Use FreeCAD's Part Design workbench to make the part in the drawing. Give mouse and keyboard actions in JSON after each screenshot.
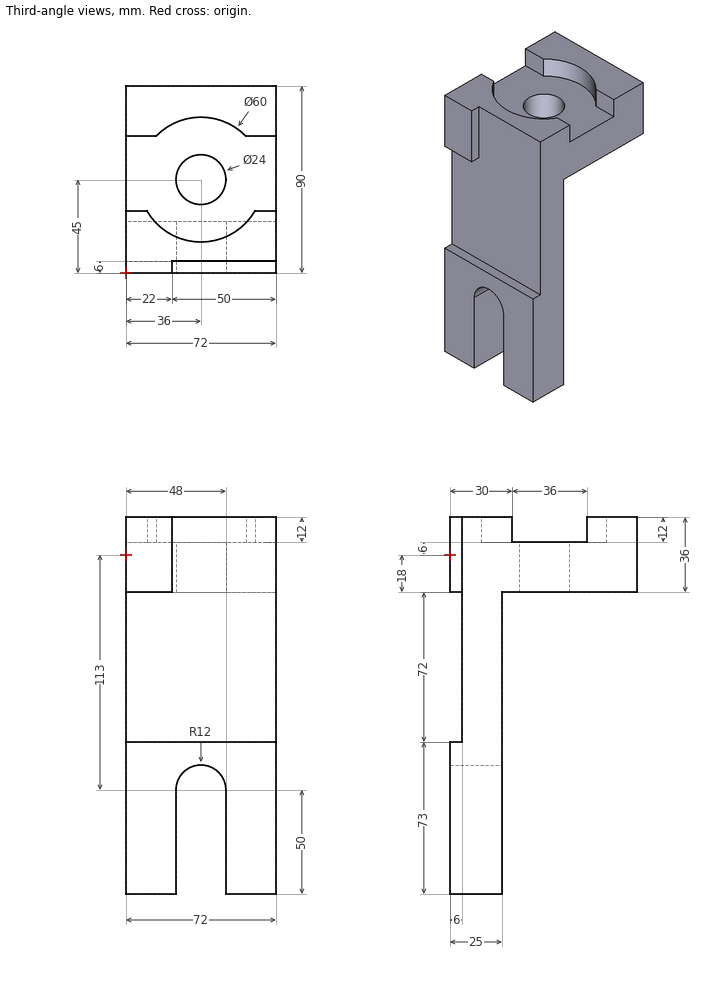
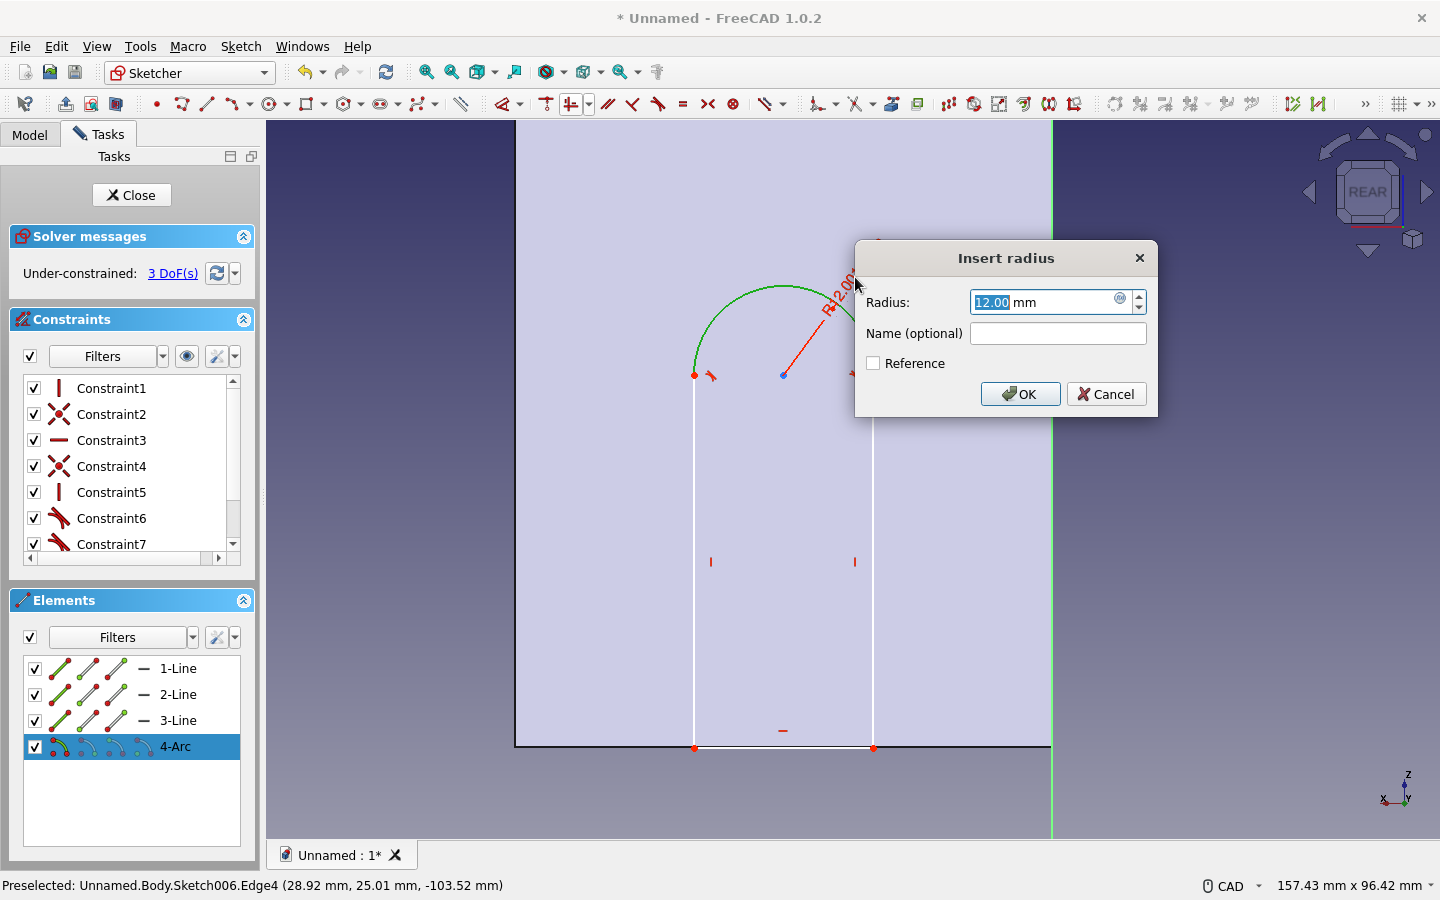
{"action": "type", "text": "12"}
{"action": "key", "text": "Return"}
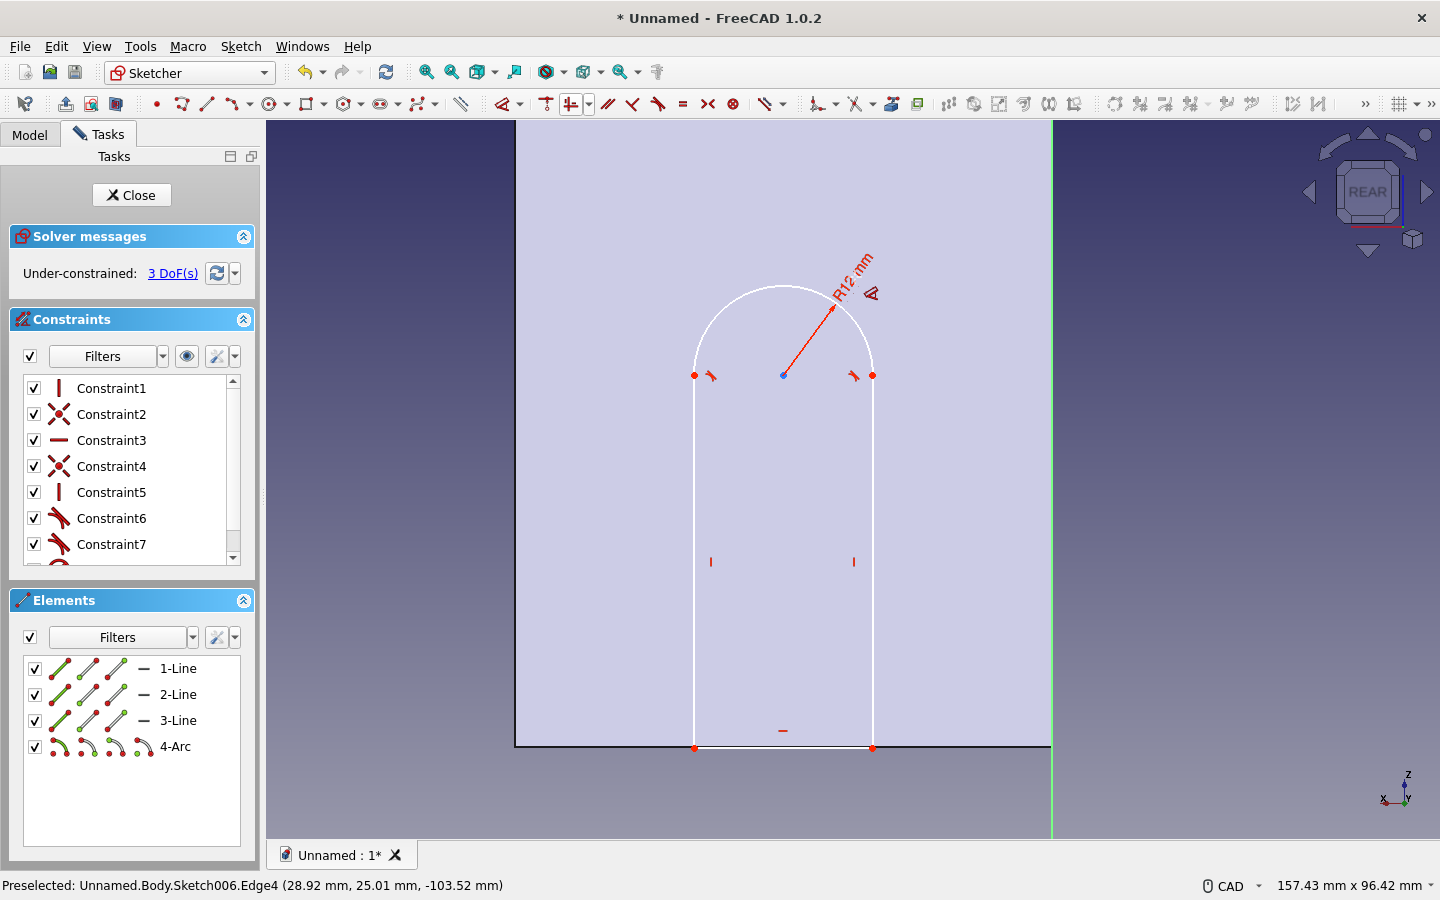
{"action": "left_click", "coordinate": [694, 487]}
{"action": "left_click", "coordinate": [660, 562]}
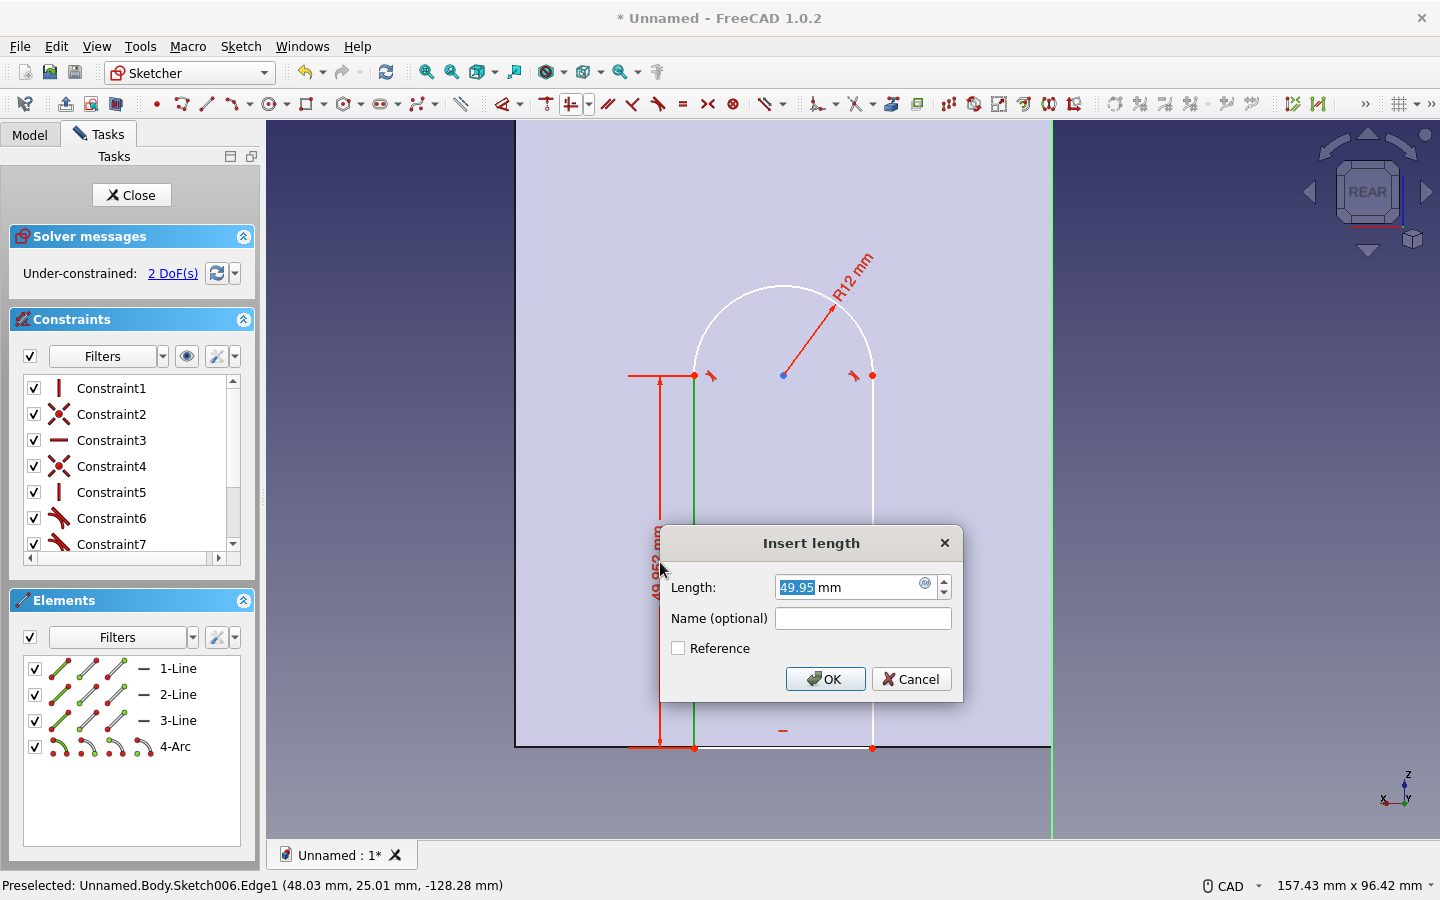
{"action": "type", "text": "50"}
{"action": "key", "text": "Return"}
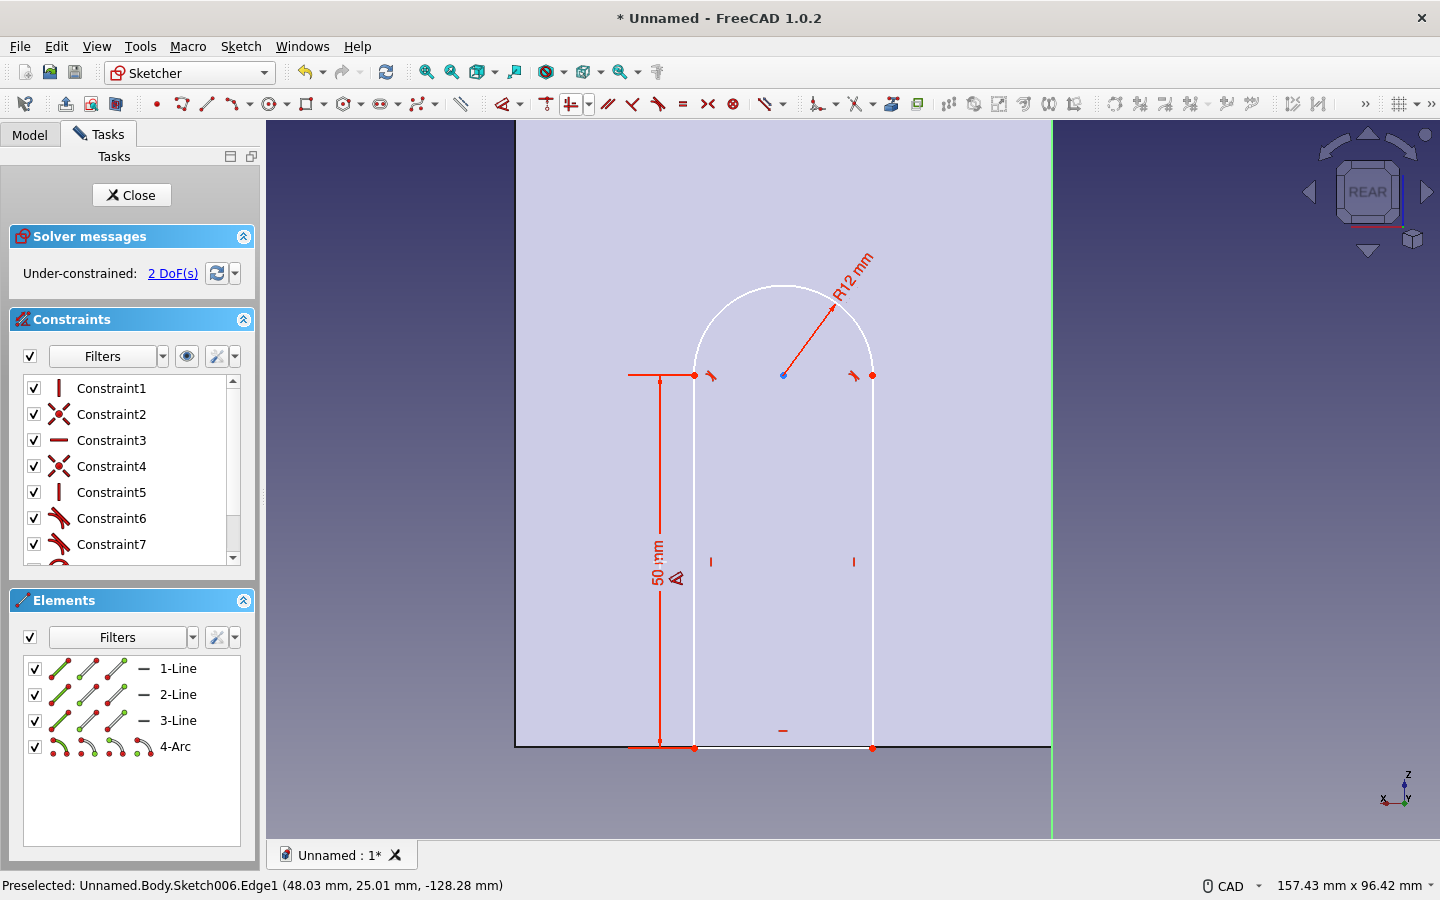
{"action": "left_click", "coordinate": [694, 375]}
{"action": "left_click", "coordinate": [791, 409]}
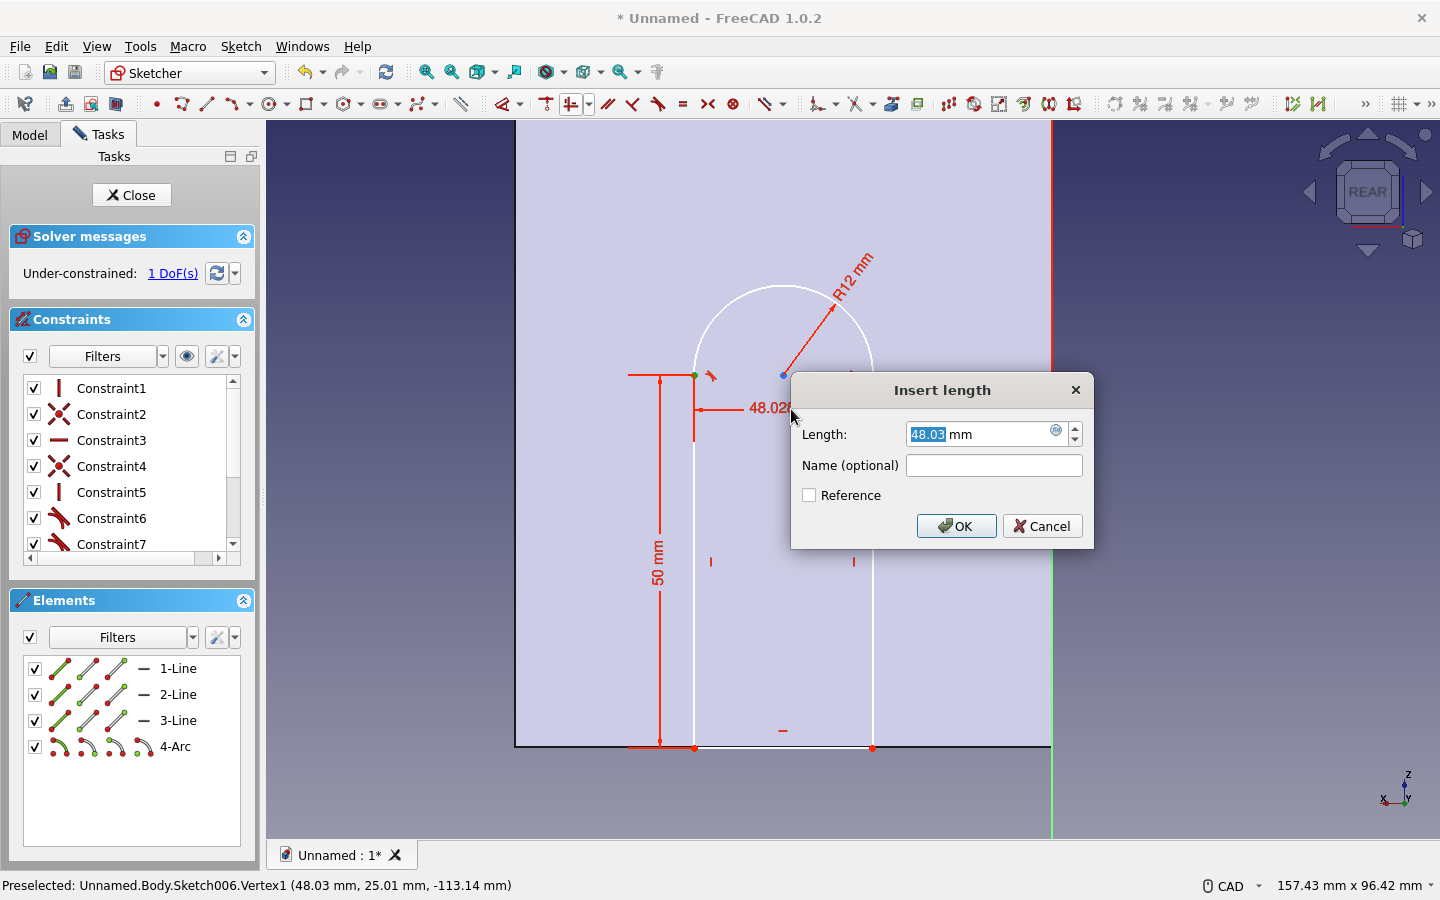
{"action": "type", "text": "48"}
{"action": "key", "text": "Return"}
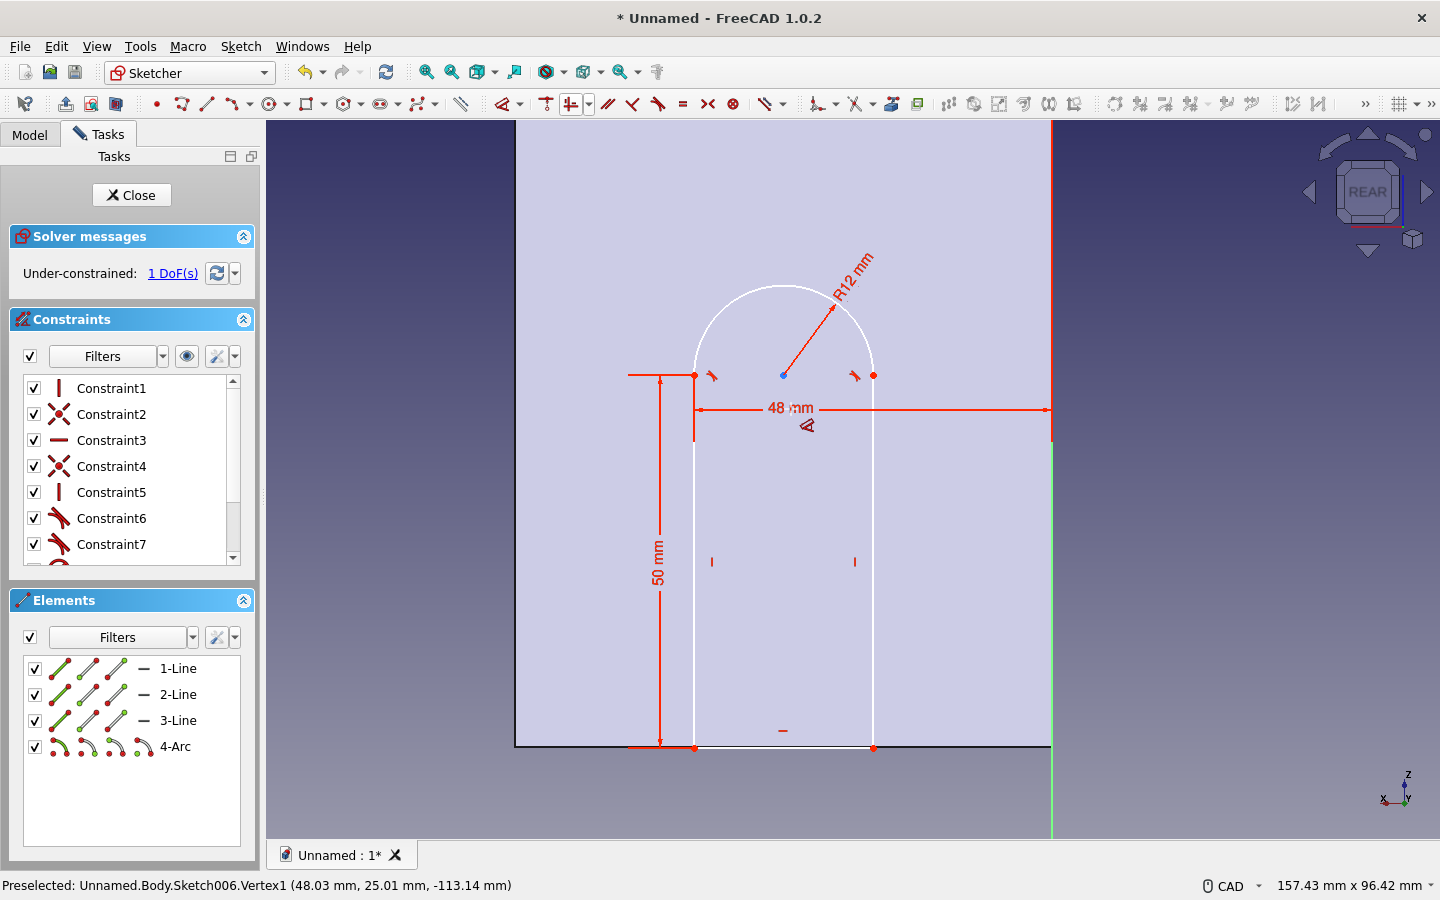
{"action": "left_click", "coordinate": [694, 375]}
{"action": "left_click", "coordinate": [1086, 262]}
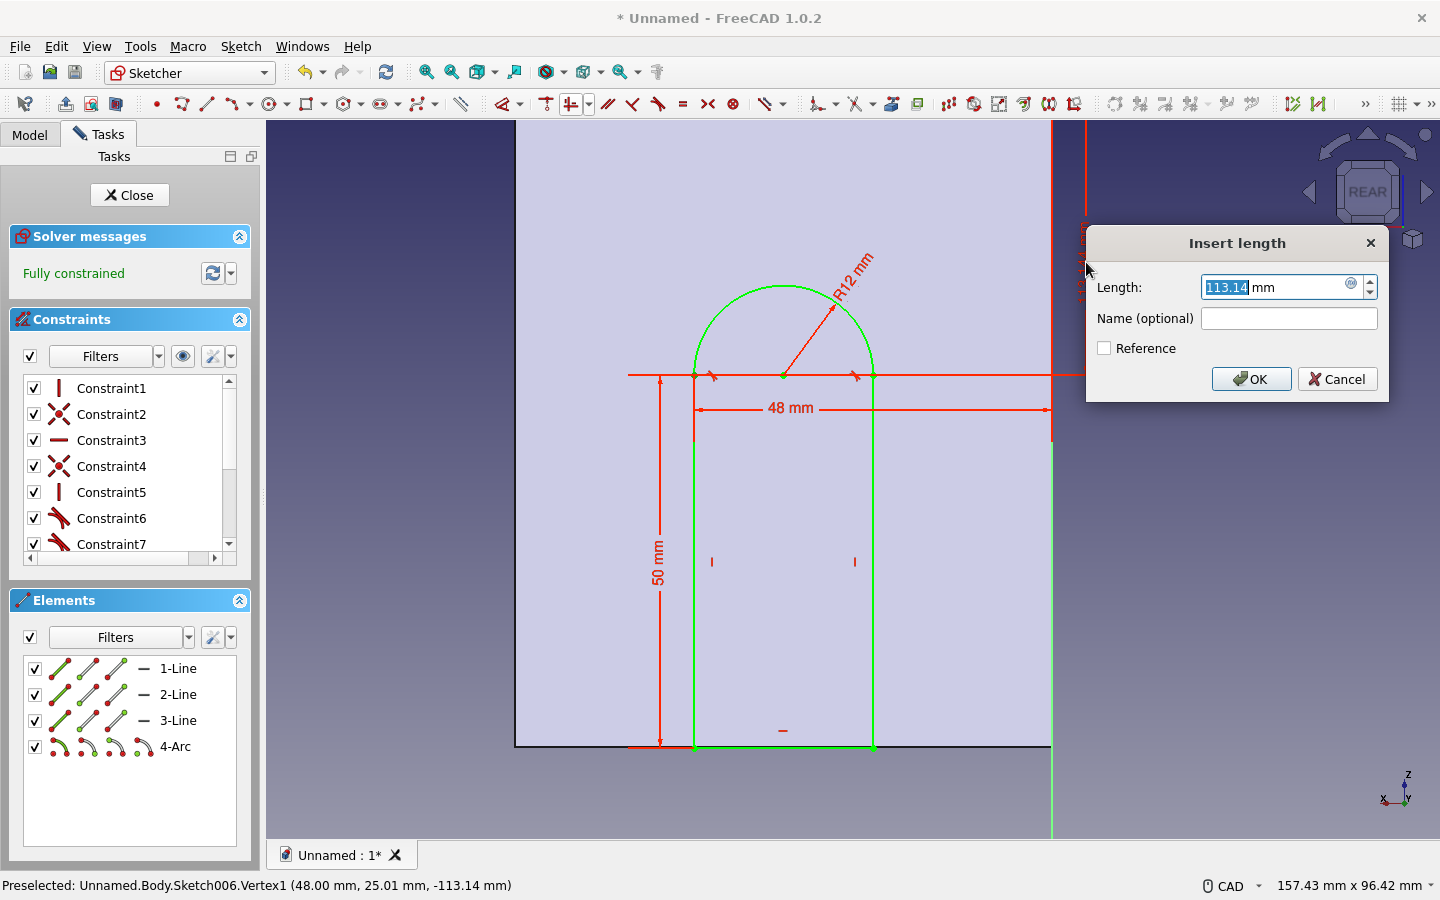
{"action": "type", "text": "113"}
{"action": "key", "text": "Return"}
{"action": "key", "text": "Escape"}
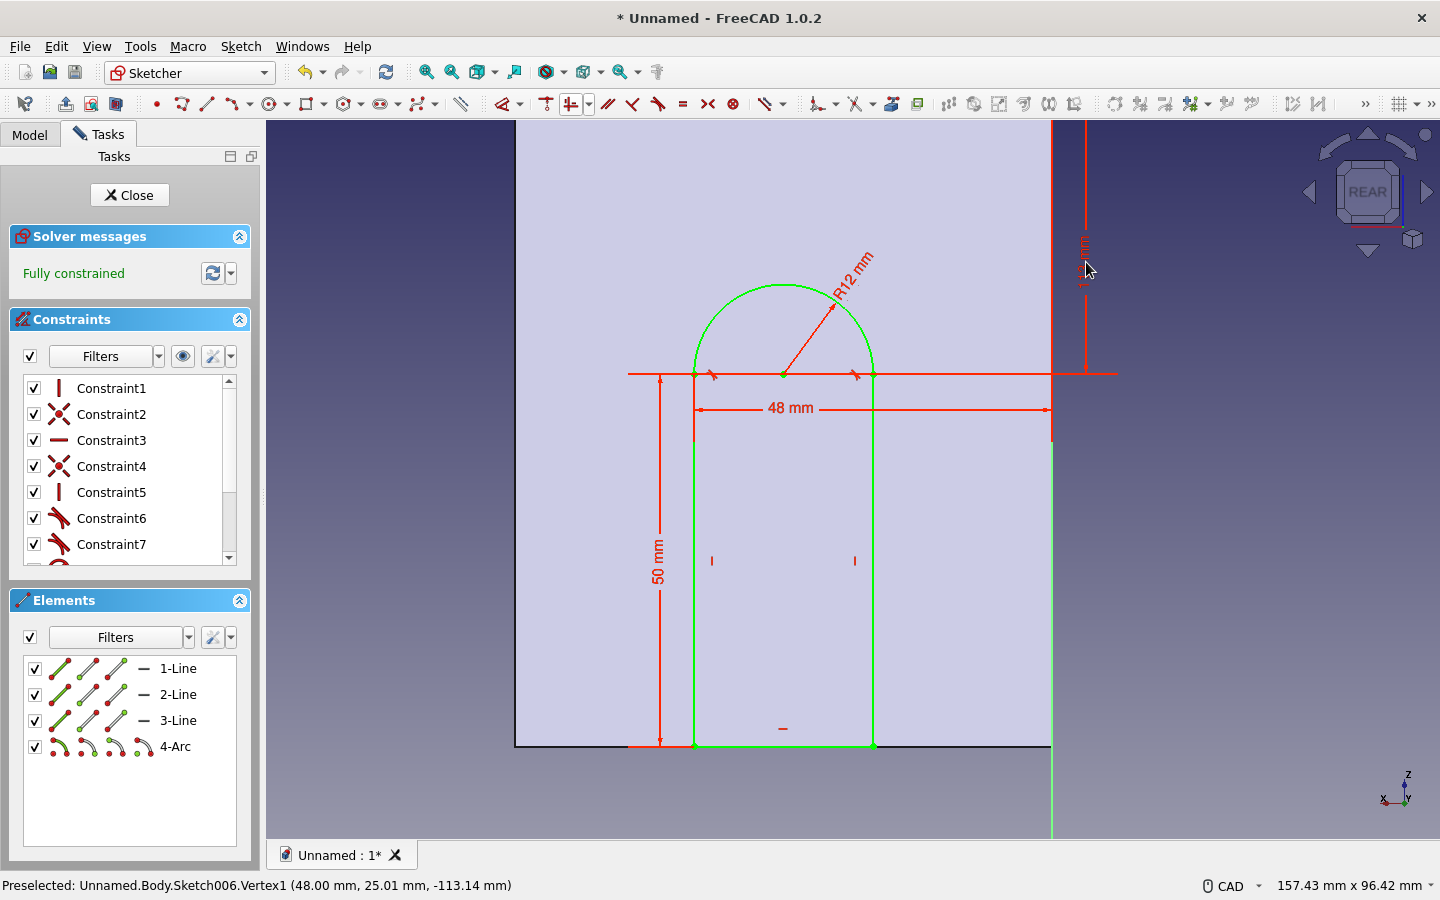
{"action": "left_click", "coordinate": [130, 195]}